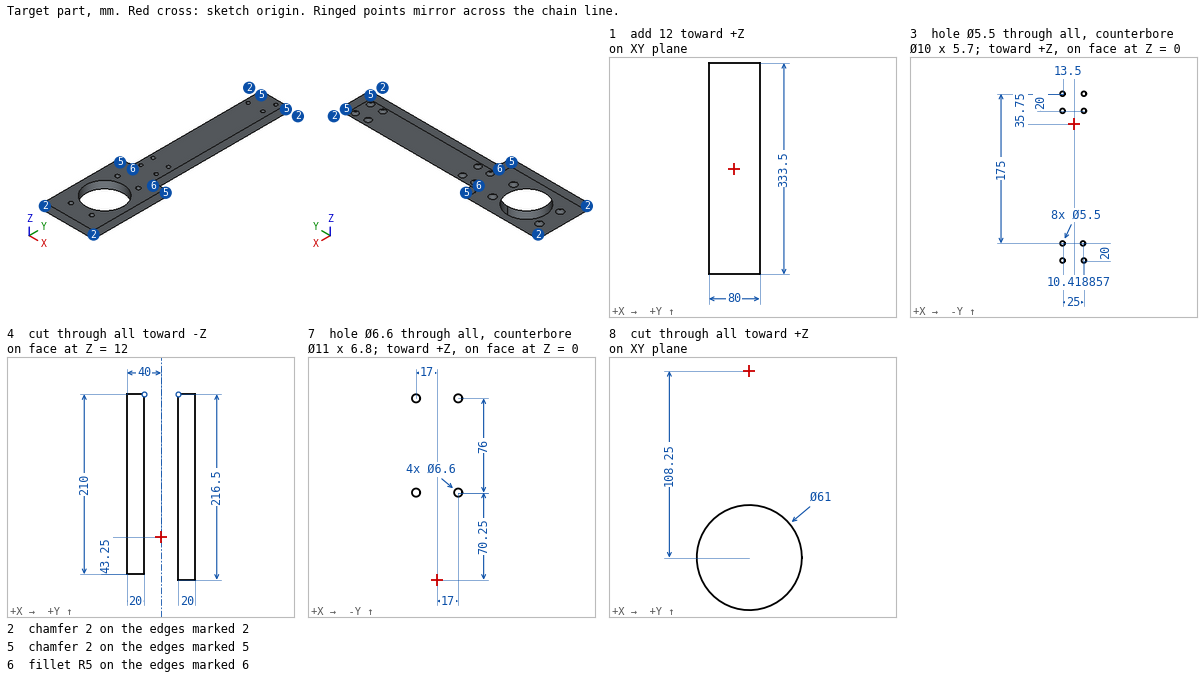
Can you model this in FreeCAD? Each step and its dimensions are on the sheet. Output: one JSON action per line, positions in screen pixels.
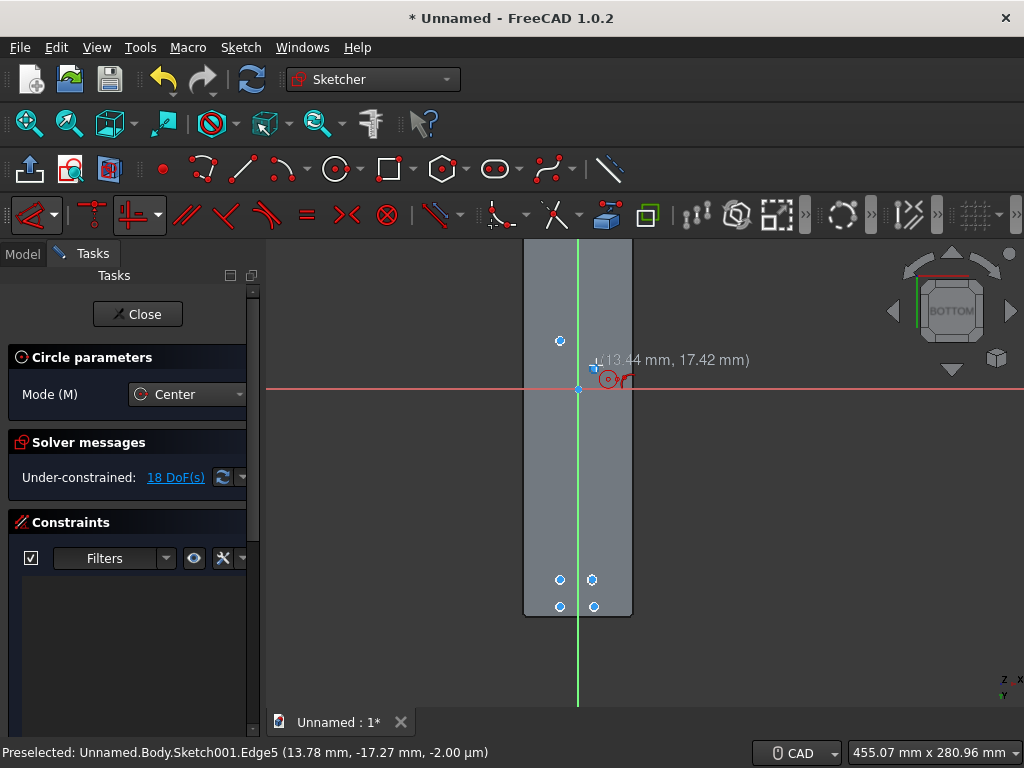
{"action": "left_click", "coordinate": [560, 368]}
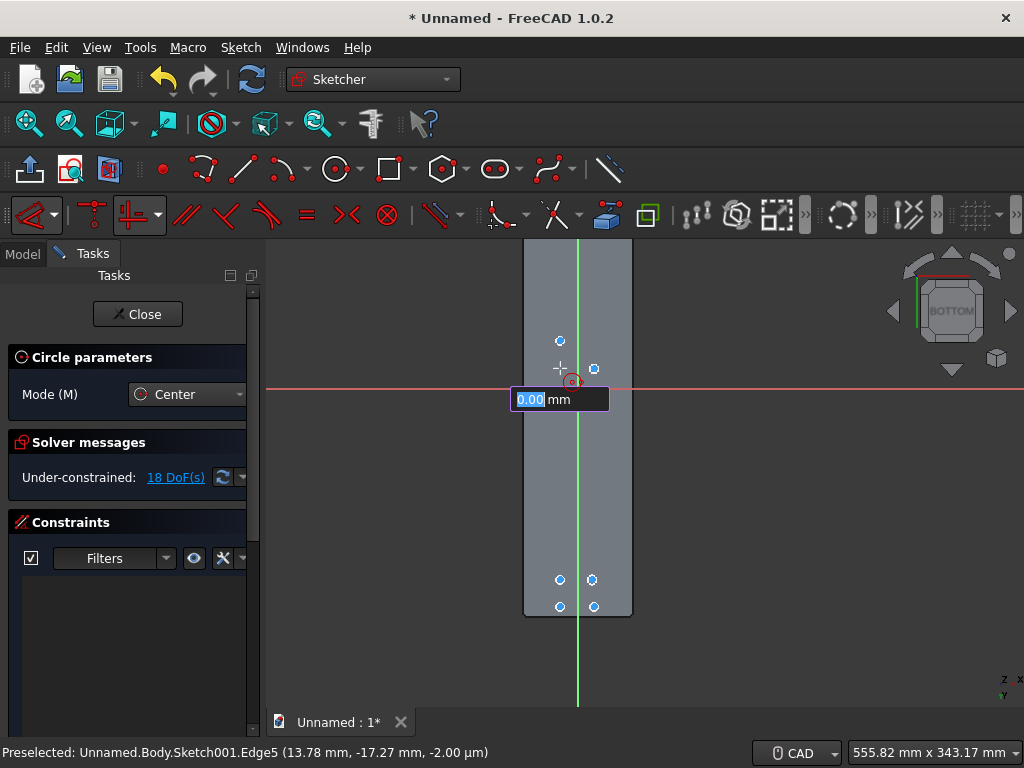
{"action": "scroll", "coordinate": [562, 365], "scroll_direction": "up", "scroll_amount": 8}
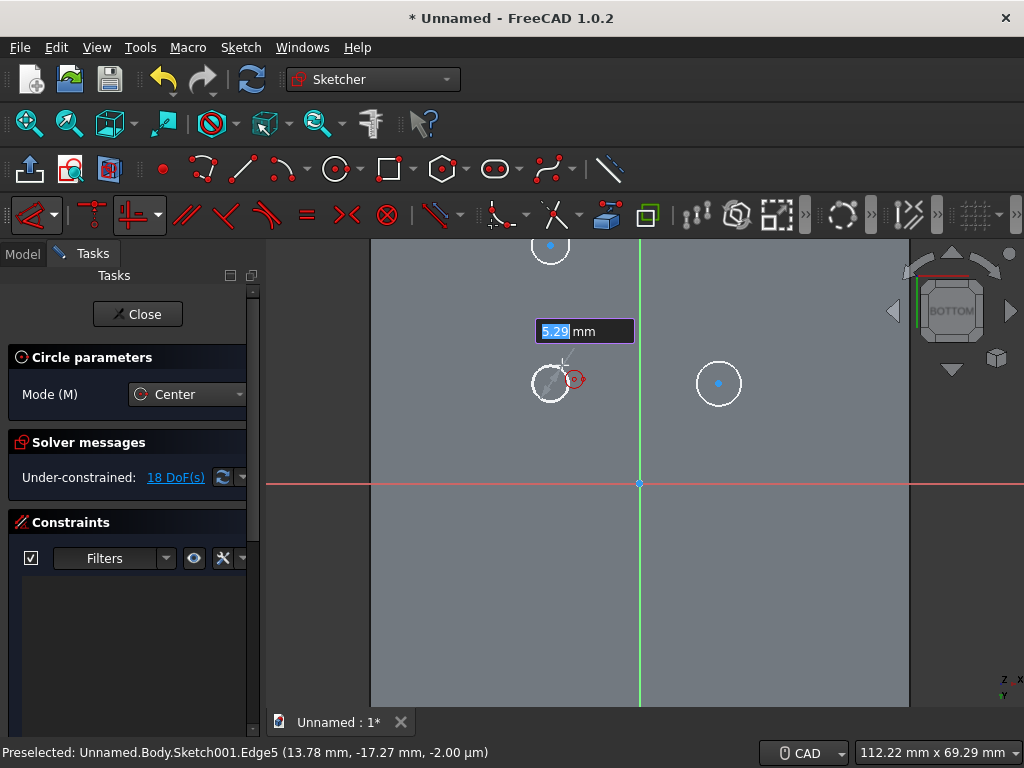
{"action": "left_click", "coordinate": [562, 364]}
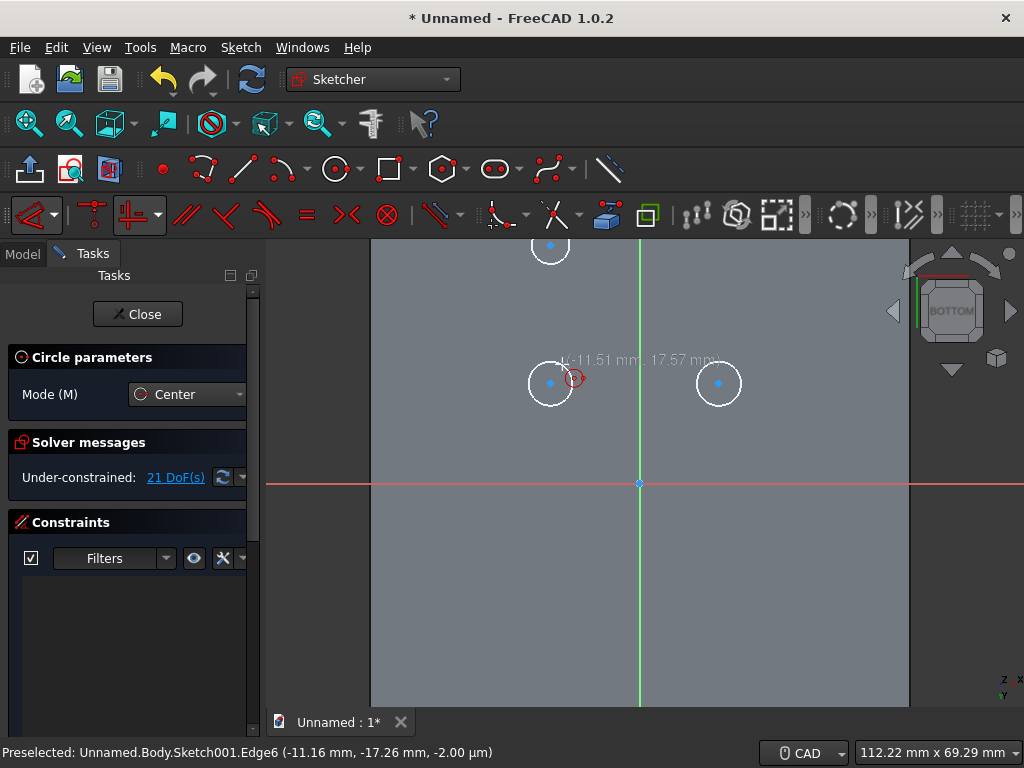
{"action": "scroll", "coordinate": [562, 365], "scroll_direction": "down", "scroll_amount": 8}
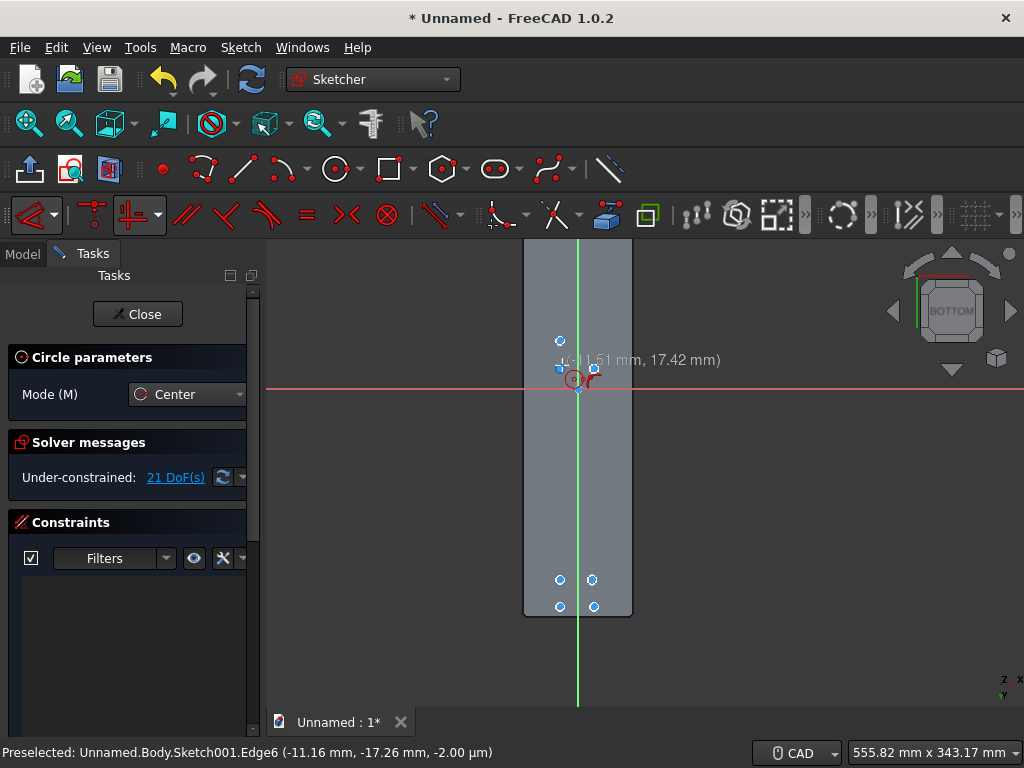
{"action": "scroll", "coordinate": [594, 340], "scroll_direction": "up", "scroll_amount": 9}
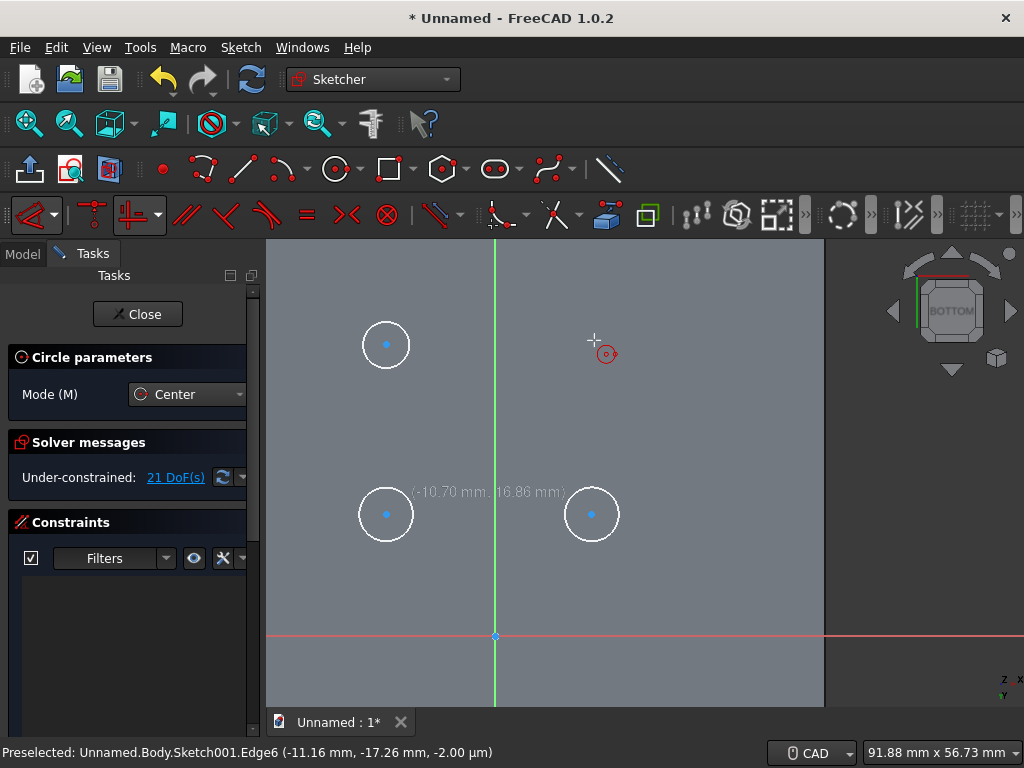
{"action": "scroll", "coordinate": [594, 340], "scroll_direction": "down", "scroll_amount": 9}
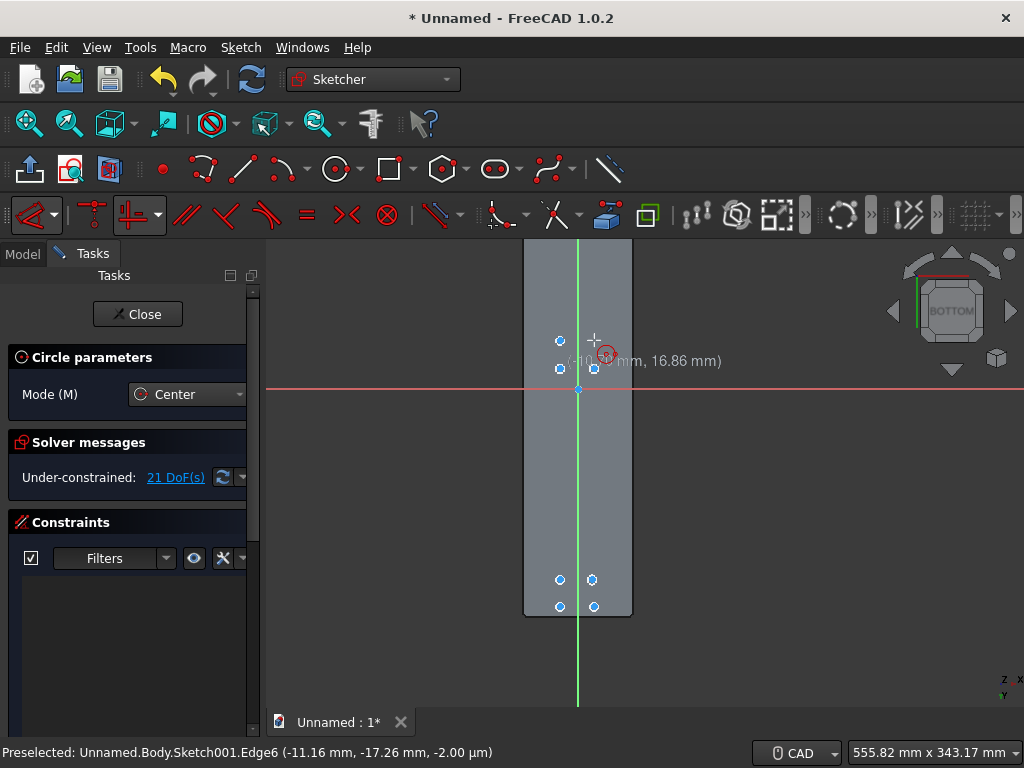
{"action": "left_click", "coordinate": [594, 340]}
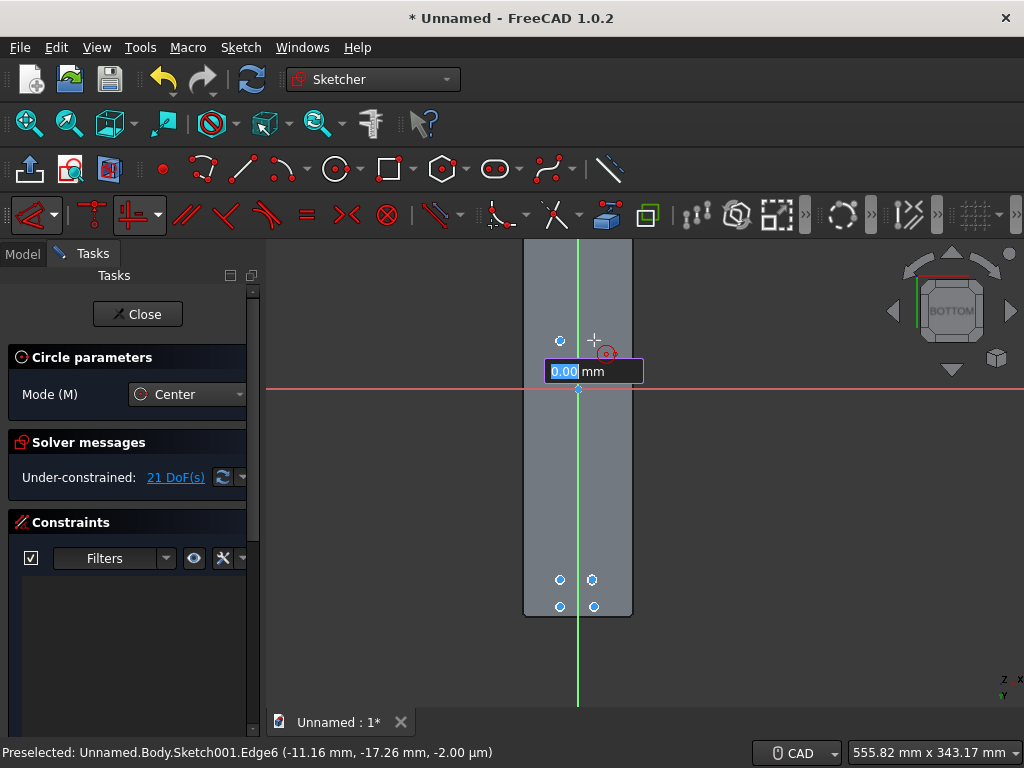
{"action": "scroll", "coordinate": [596, 338], "scroll_direction": "up", "scroll_amount": 8}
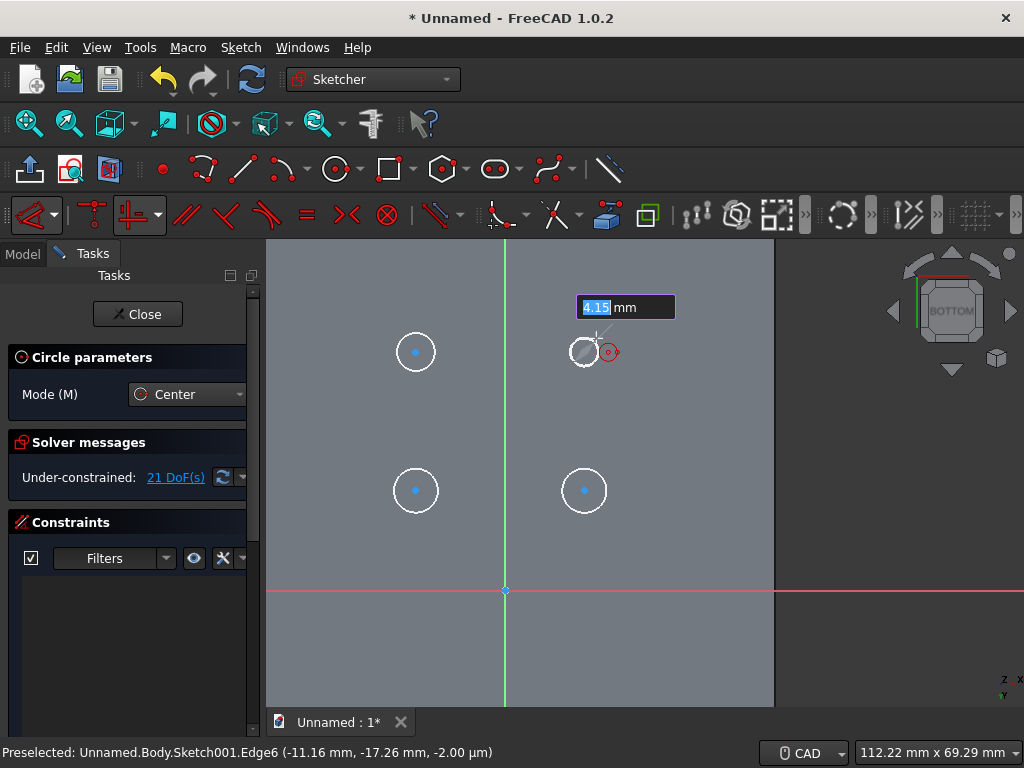
{"action": "left_click", "coordinate": [596, 336]}
{"action": "key", "text": "Escape"}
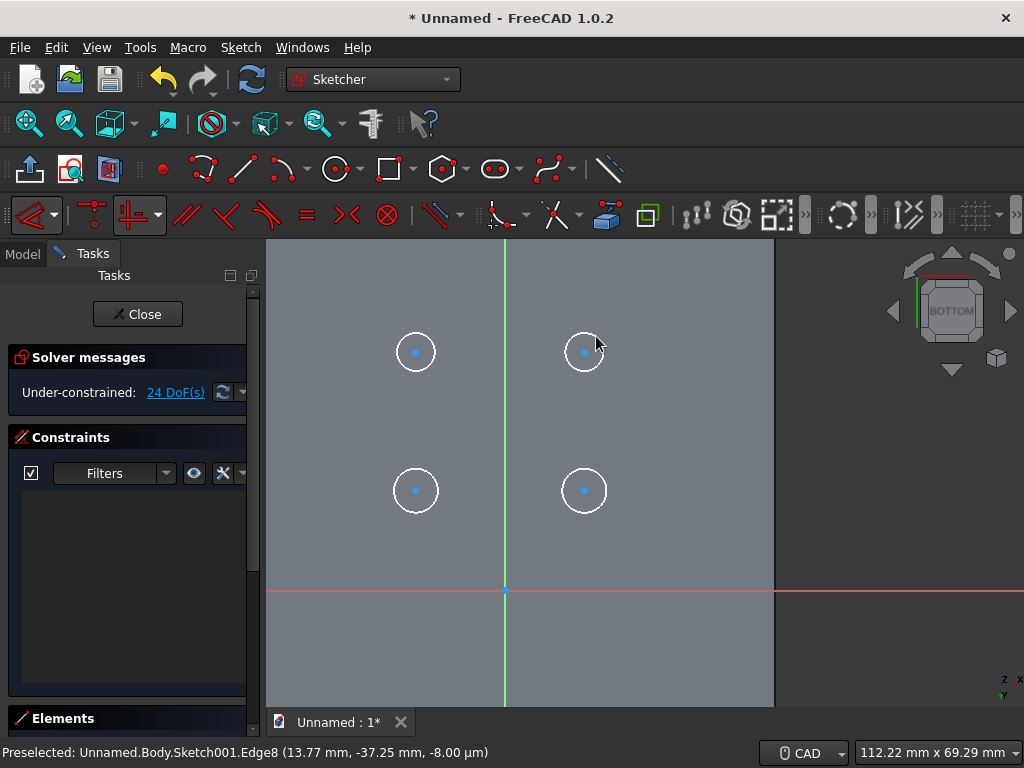
{"action": "left_click", "coordinate": [429, 339]}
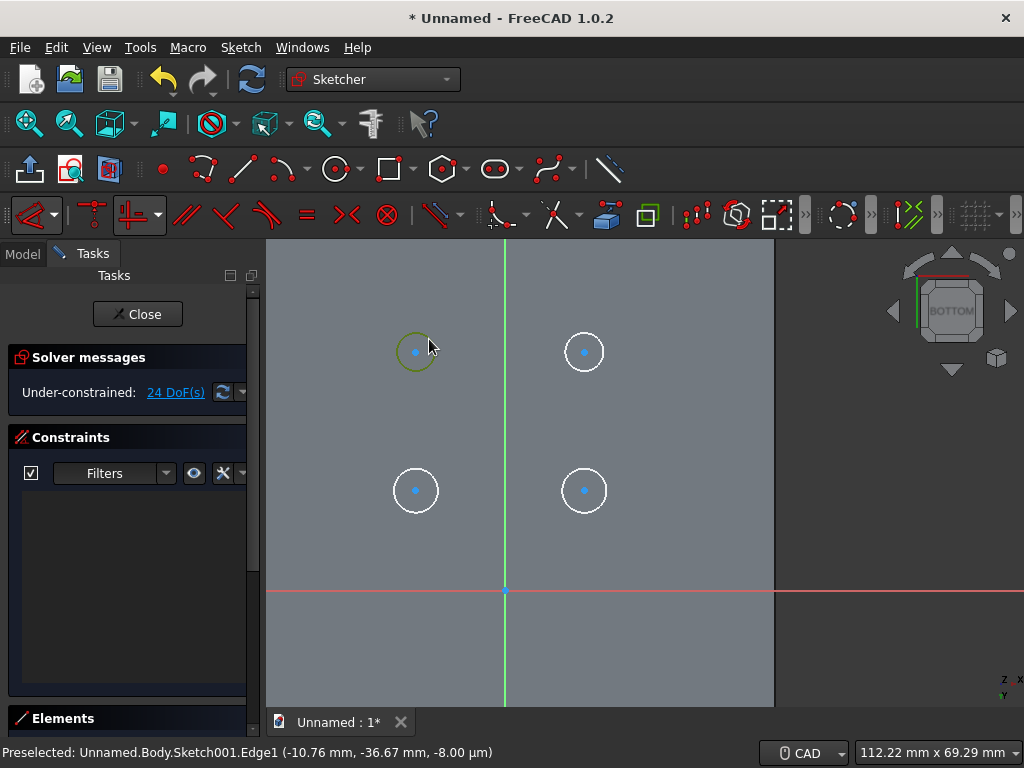
{"action": "scroll", "coordinate": [596, 338], "scroll_direction": "down", "scroll_amount": 8}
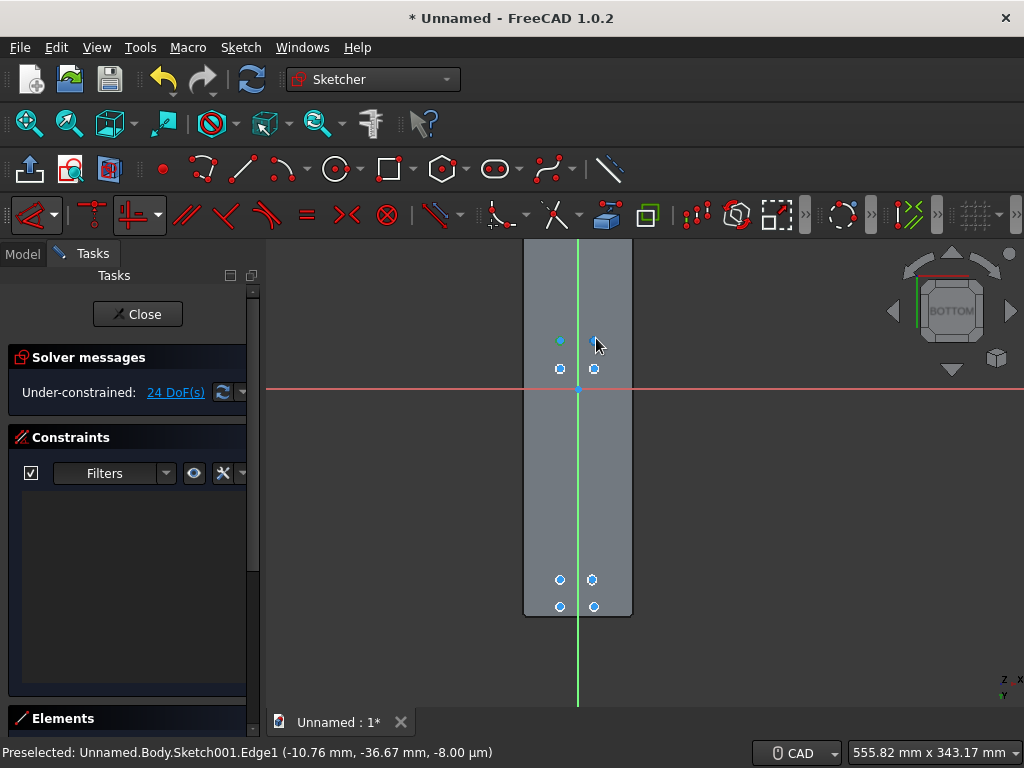
{"action": "scroll", "coordinate": [563, 577], "scroll_direction": "up", "scroll_amount": 7}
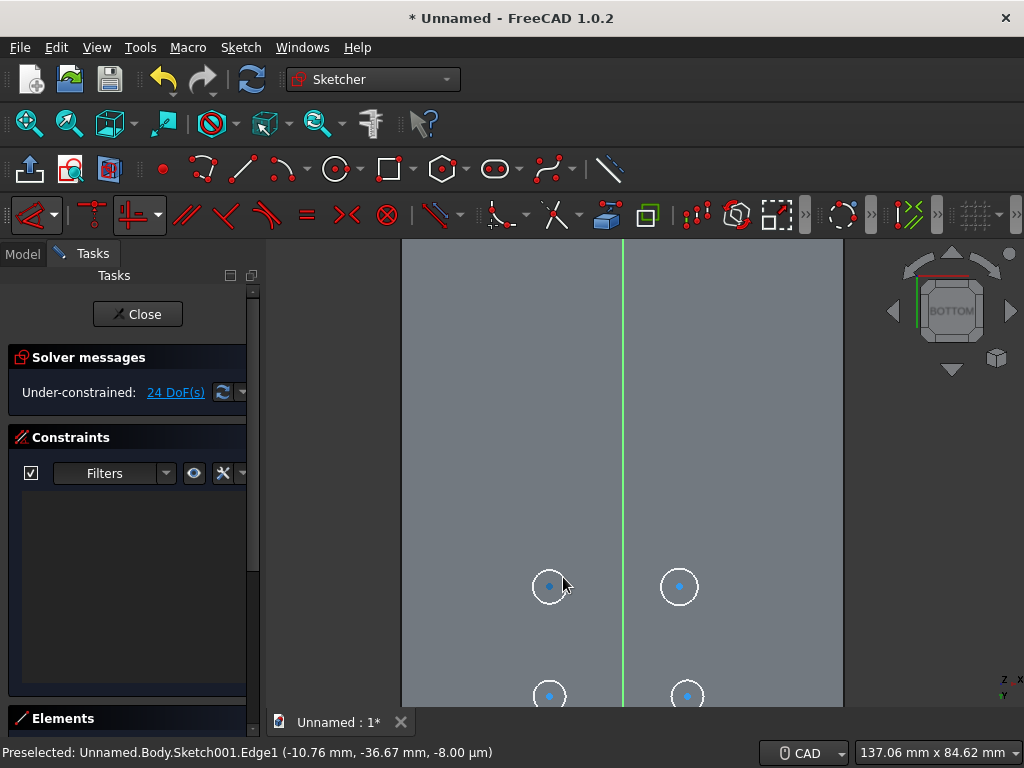
{"action": "left_click", "coordinate": [561, 575]}